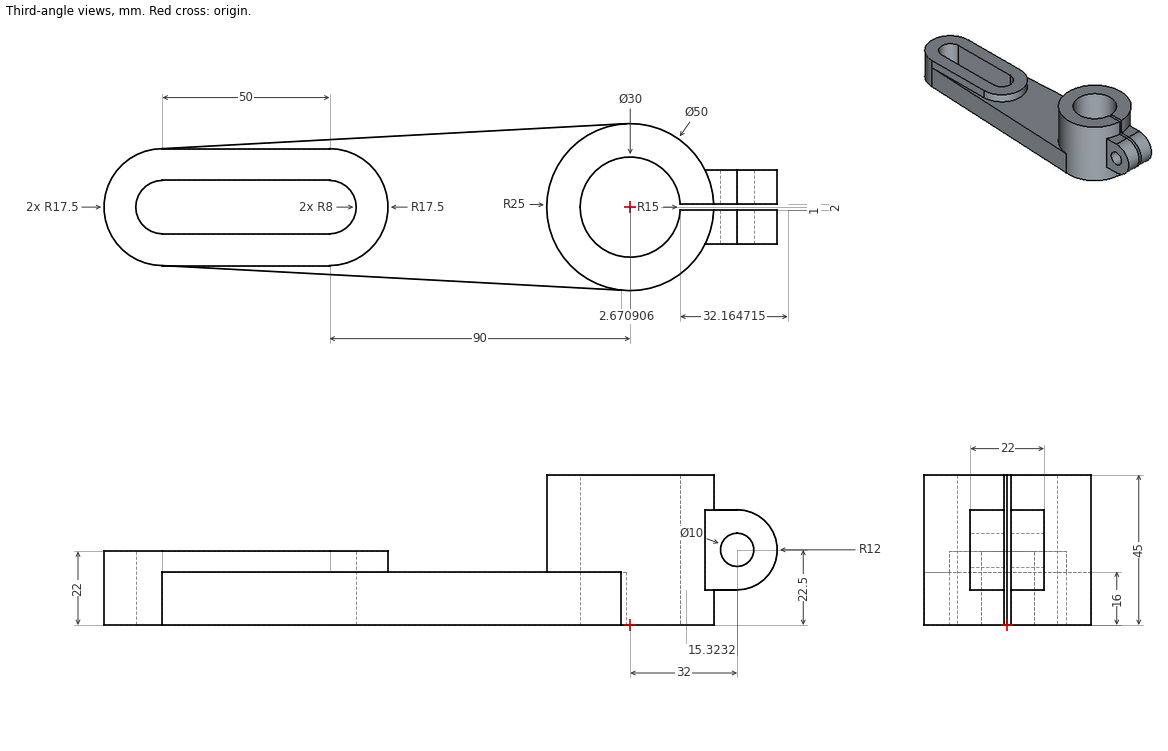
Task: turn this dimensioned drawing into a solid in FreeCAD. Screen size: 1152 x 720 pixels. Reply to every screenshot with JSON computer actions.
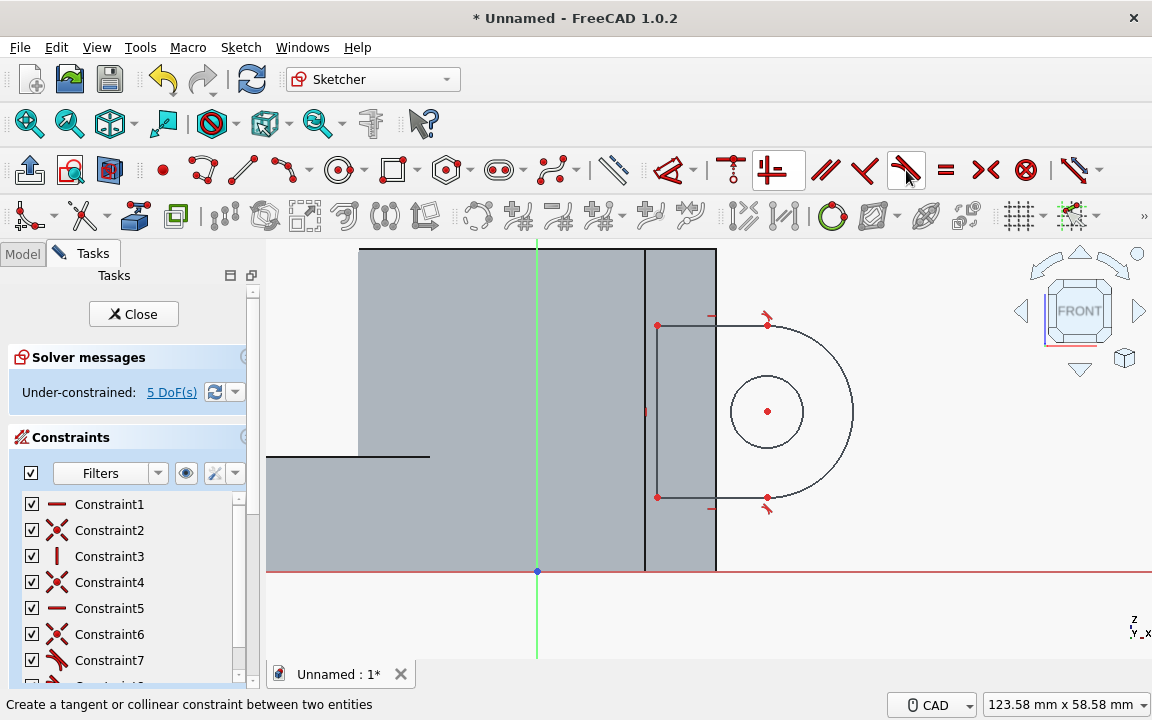
{"action": "left_click", "coordinate": [837, 463]}
{"action": "left_click", "coordinate": [863, 482]}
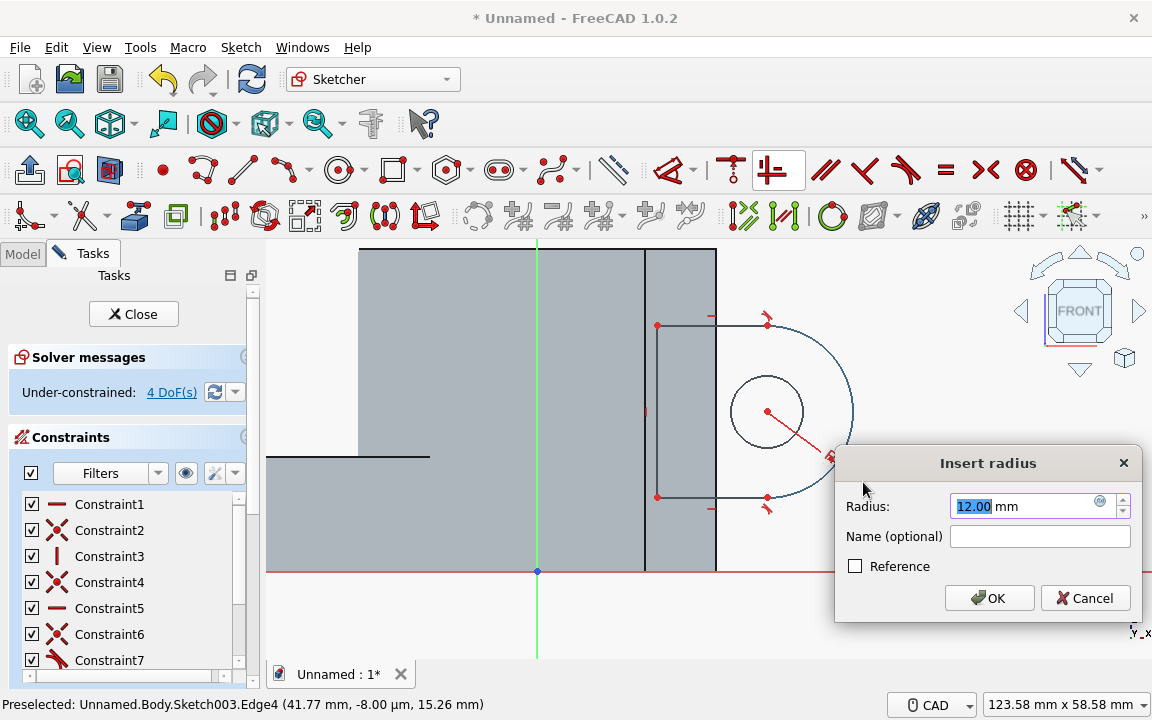
{"action": "type", "text": "12"}
{"action": "key", "text": "Return"}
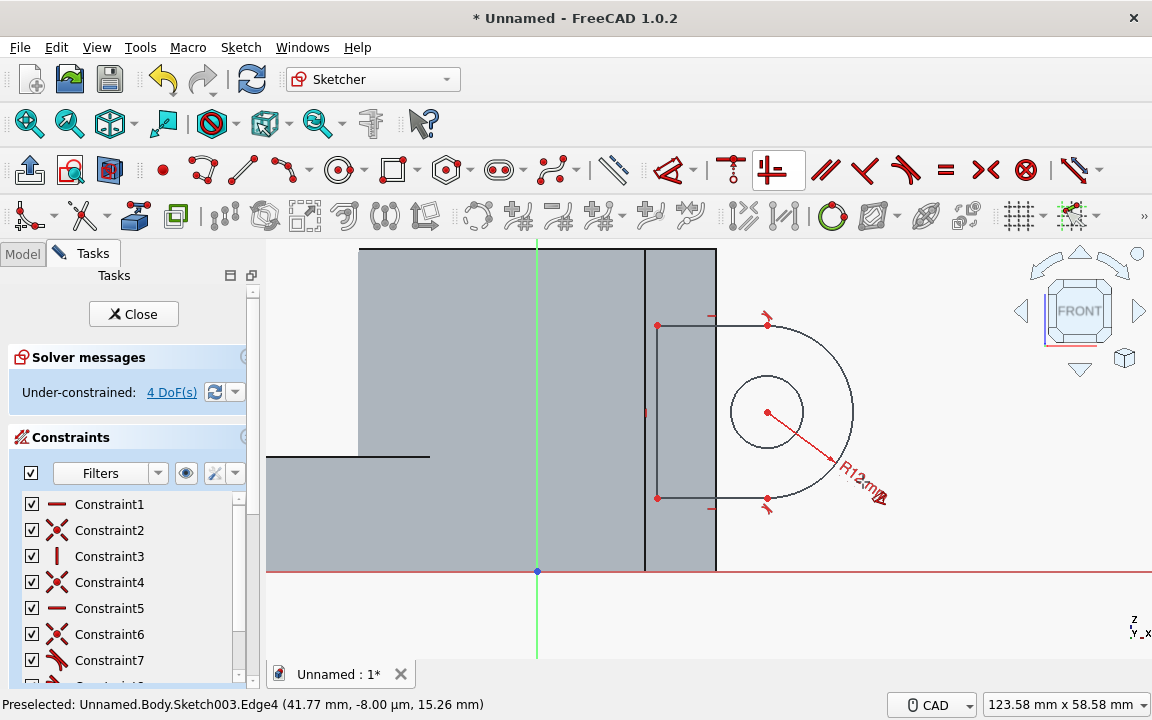
{"action": "left_click", "coordinate": [792, 386]}
{"action": "left_click", "coordinate": [814, 363]}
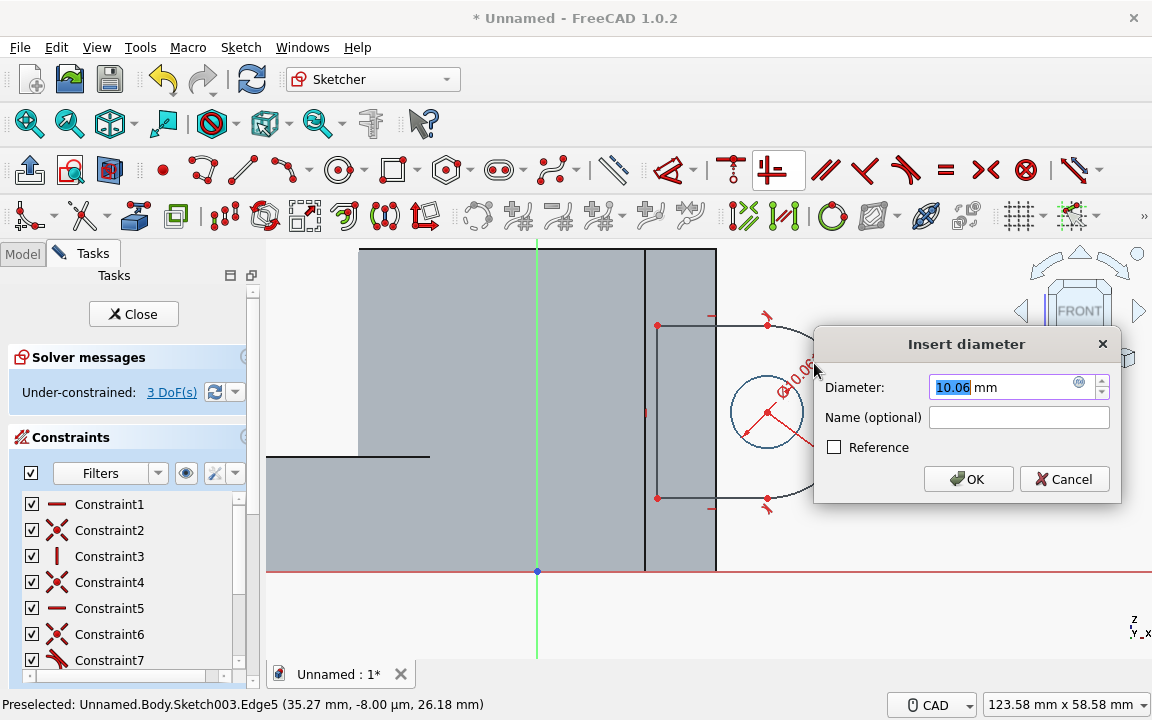
{"action": "type", "text": "10"}
{"action": "key", "text": "Return"}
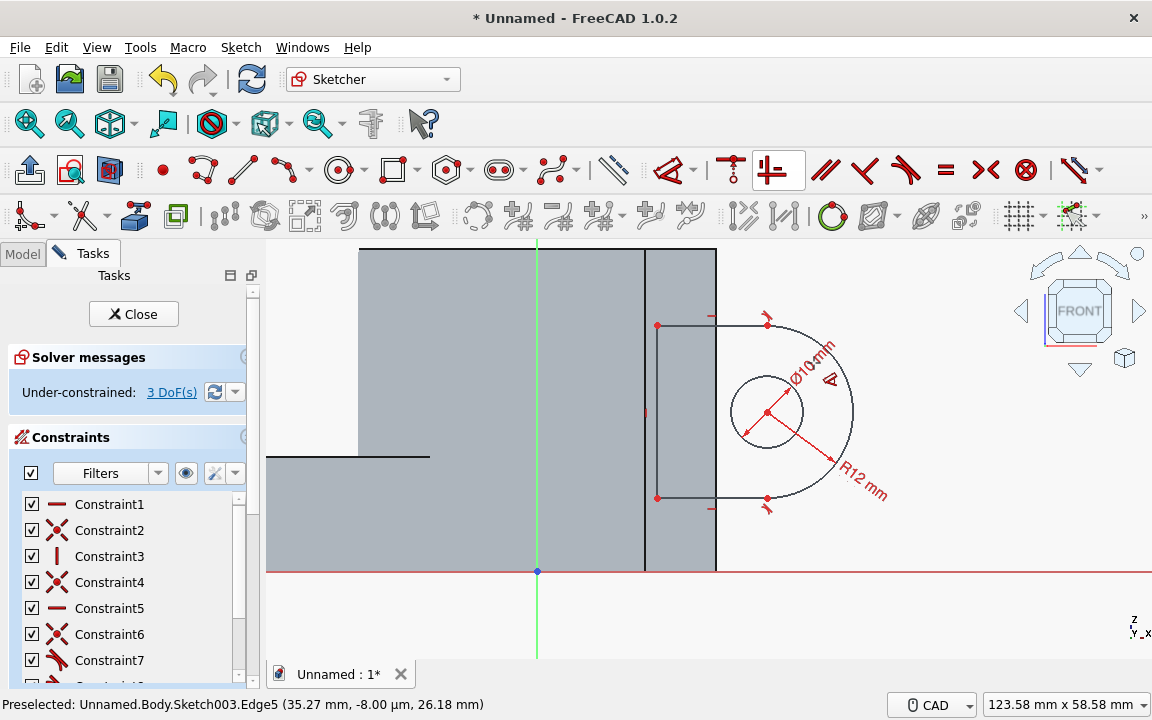
{"action": "left_click", "coordinate": [767, 412]}
{"action": "left_click", "coordinate": [652, 606]}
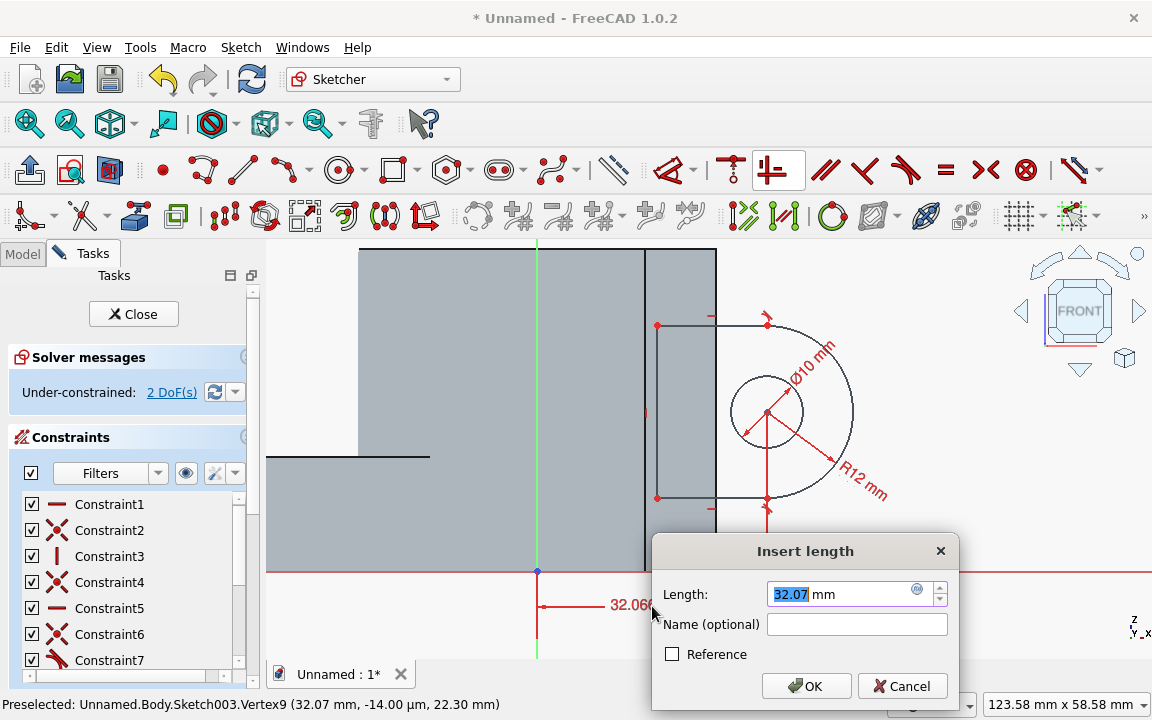
{"action": "type", "text": "32"}
{"action": "key", "text": "Return"}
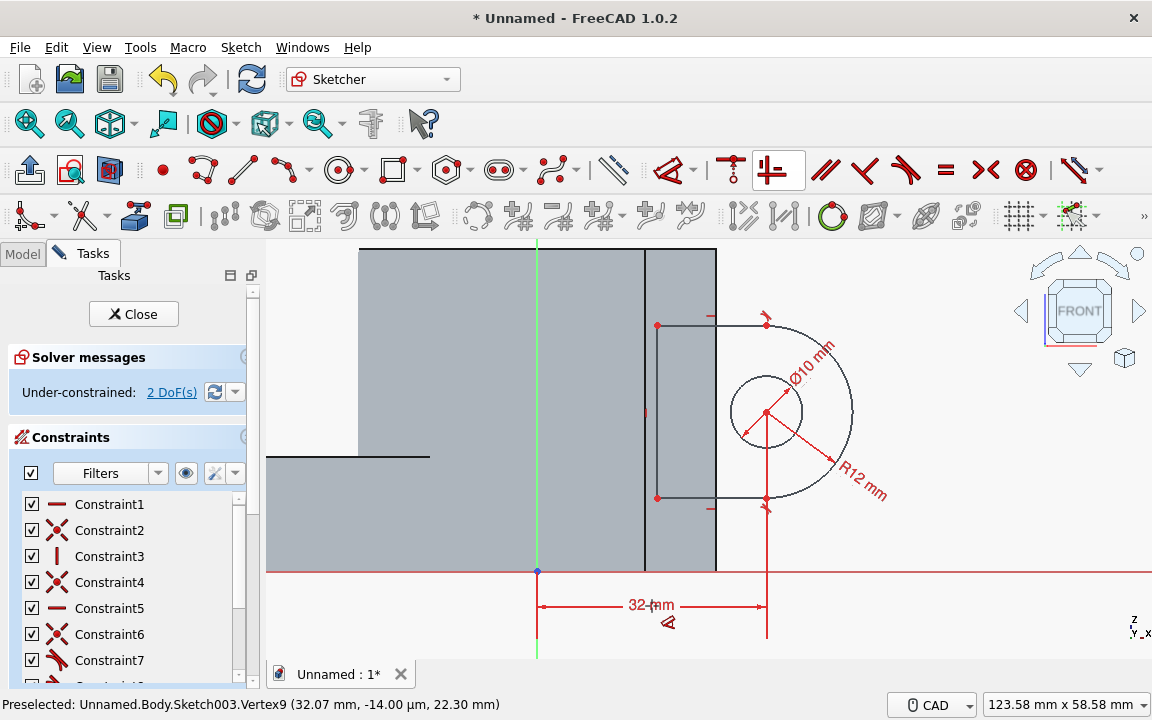
{"action": "left_click", "coordinate": [767, 412]}
{"action": "left_click", "coordinate": [503, 492]}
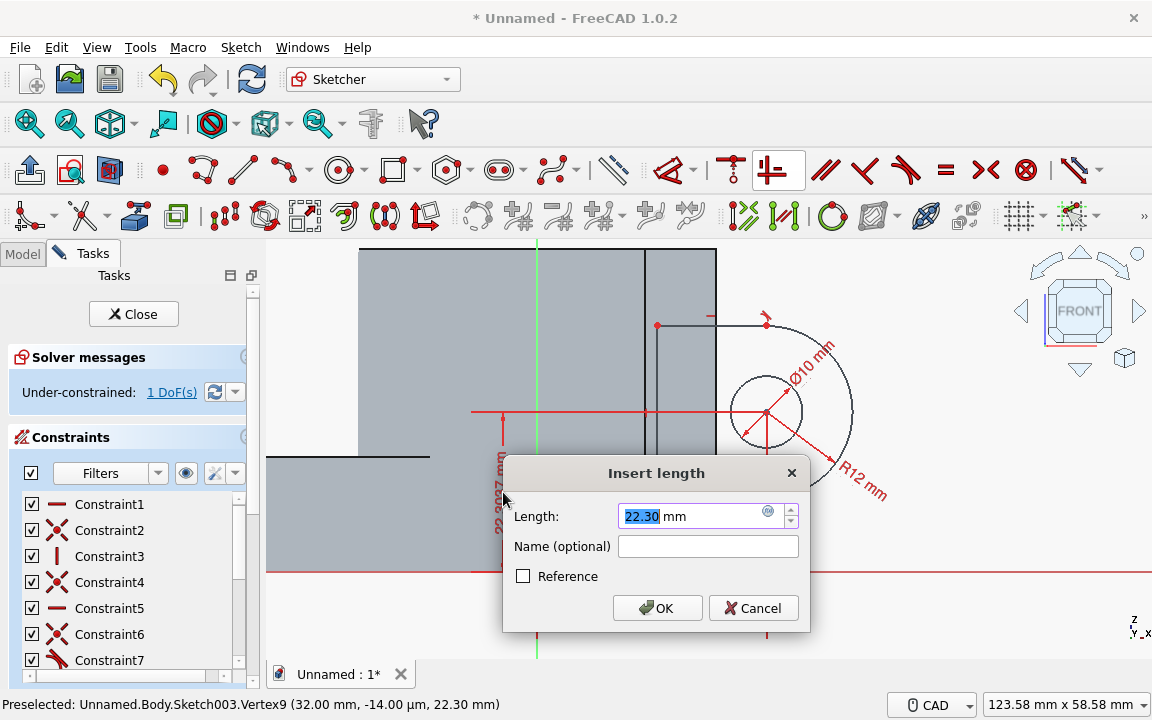
{"action": "type", "text": "22.5"}
{"action": "key", "text": "Return"}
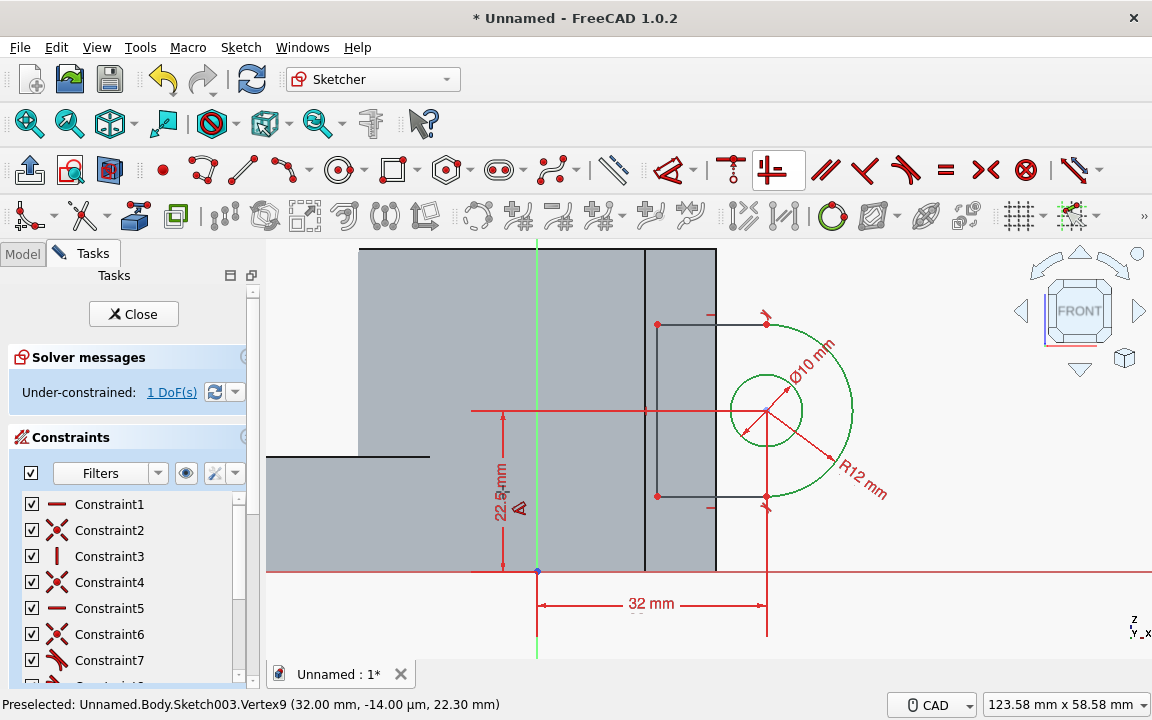
{"action": "left_click", "coordinate": [734, 497]}
{"action": "left_click", "coordinate": [712, 531]}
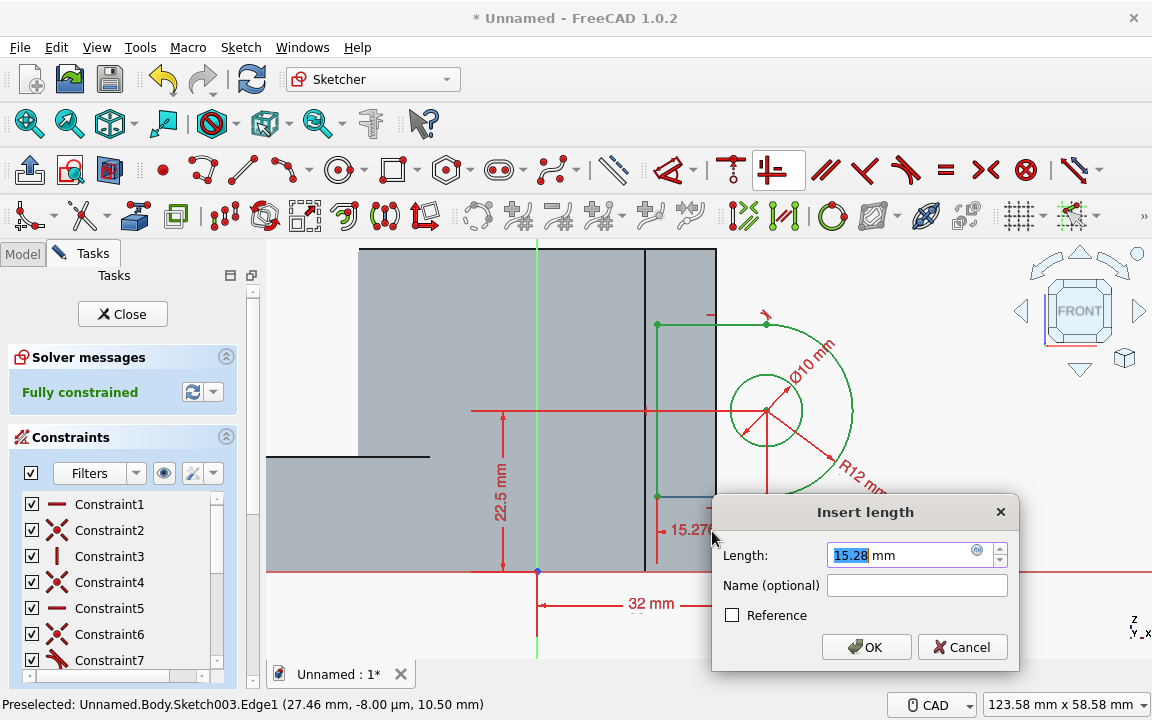
{"action": "type", "text": "15.3232"}
{"action": "key", "text": "Return"}
{"action": "key", "text": "Escape"}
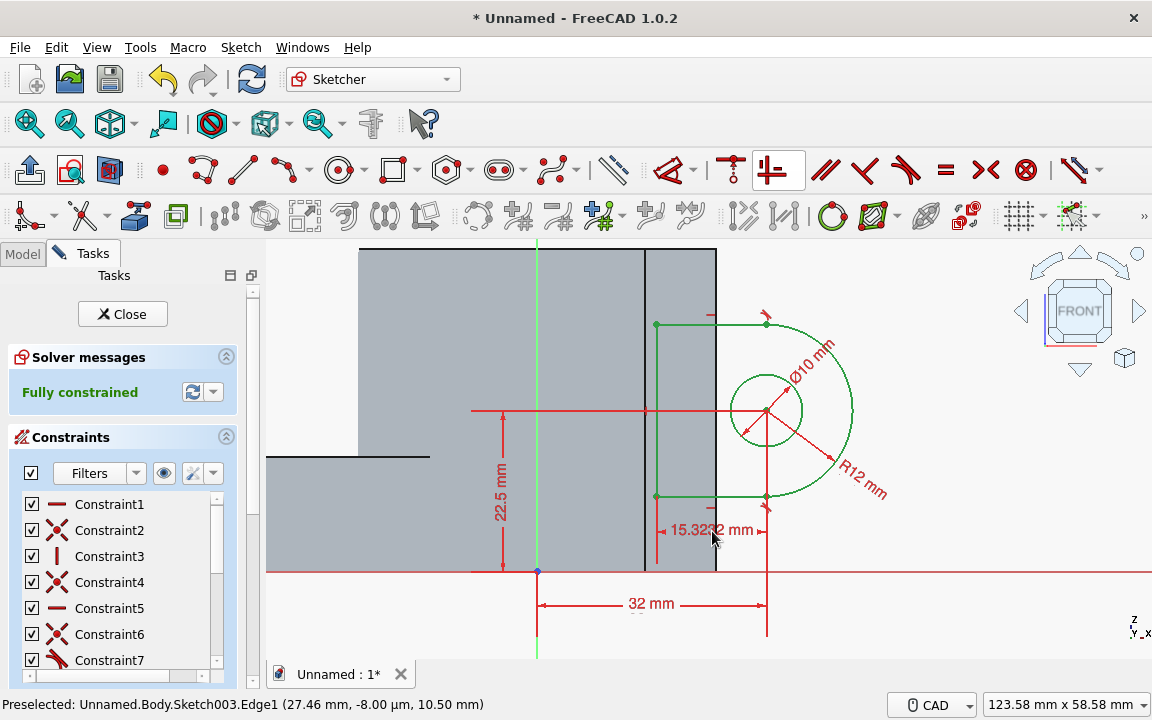
{"action": "left_click", "coordinate": [123, 314]}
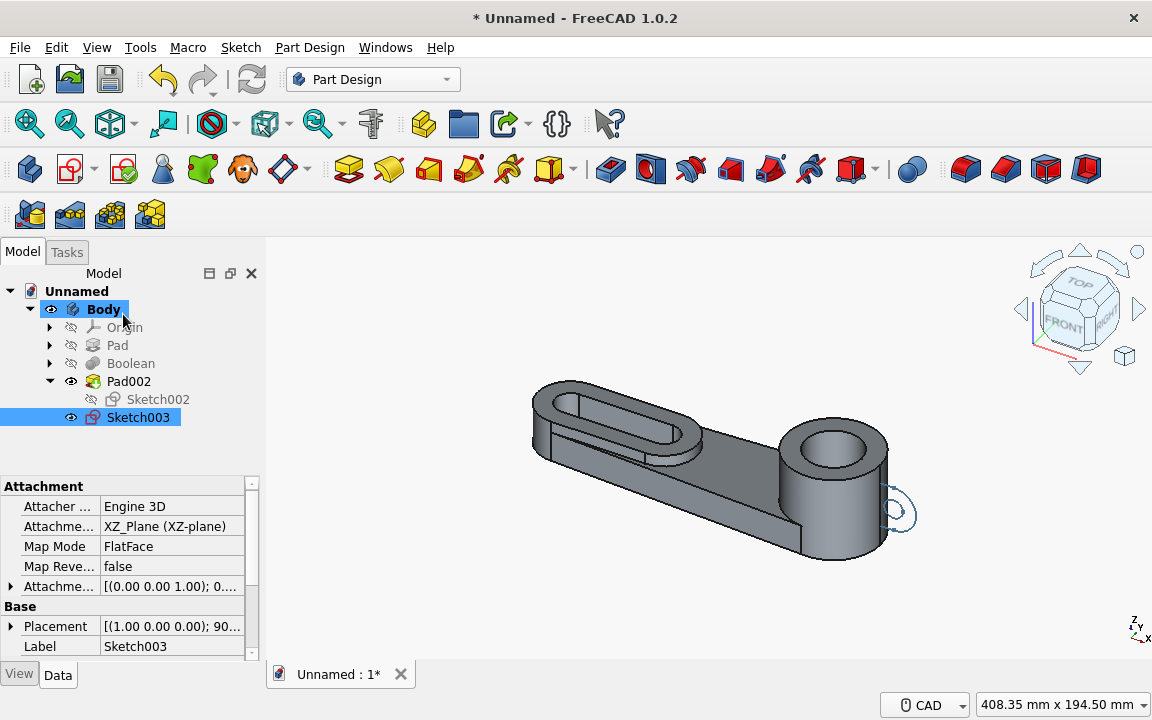
{"action": "left_click", "coordinate": [350, 170]}